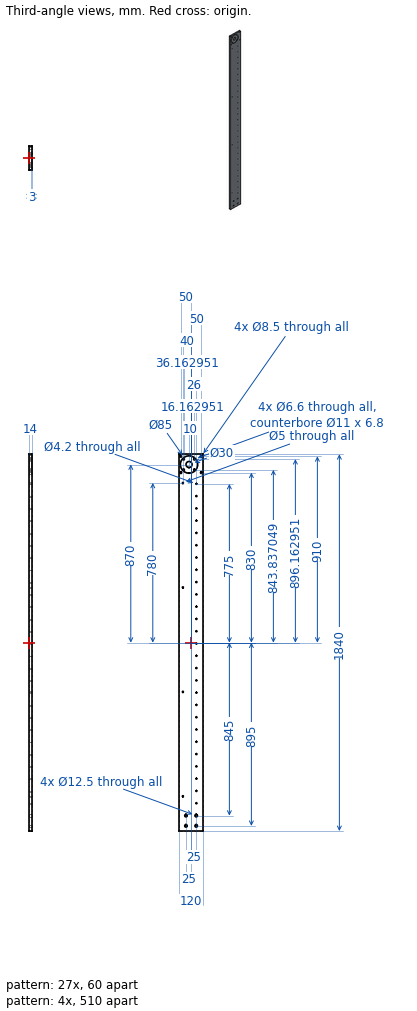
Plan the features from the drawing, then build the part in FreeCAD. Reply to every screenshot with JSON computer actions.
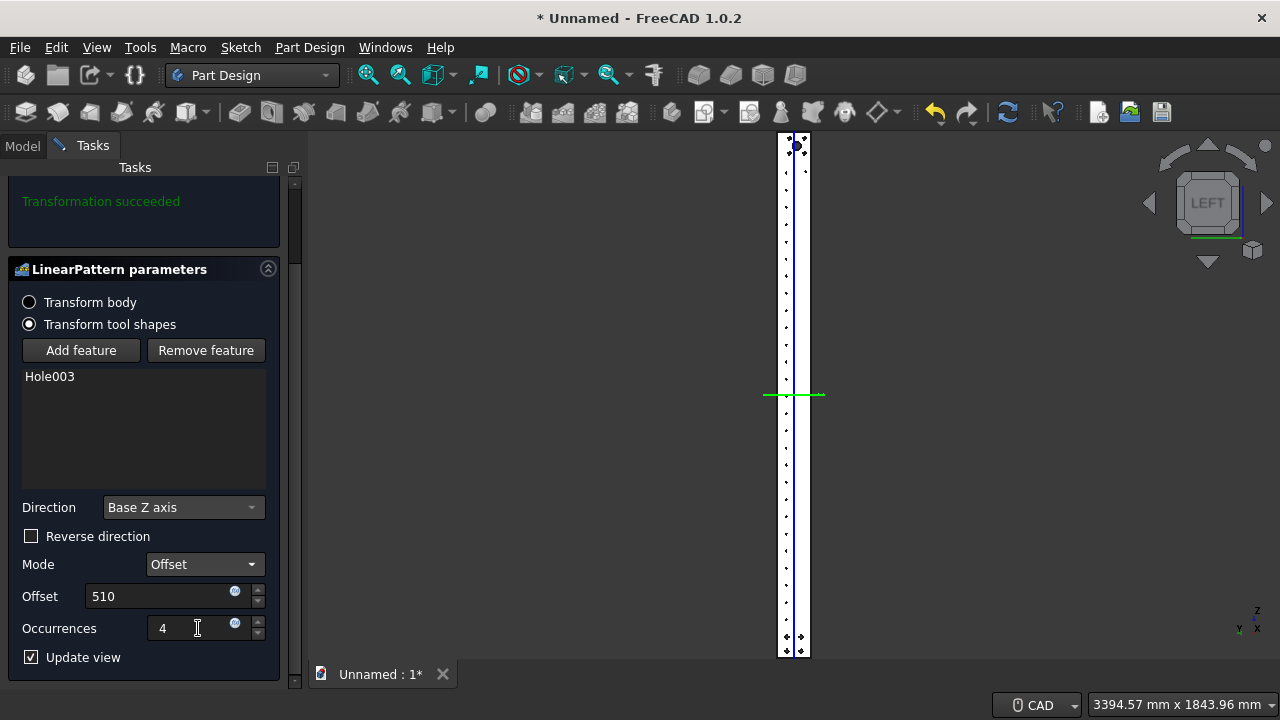
{"action": "left_click", "coordinate": [30, 536]}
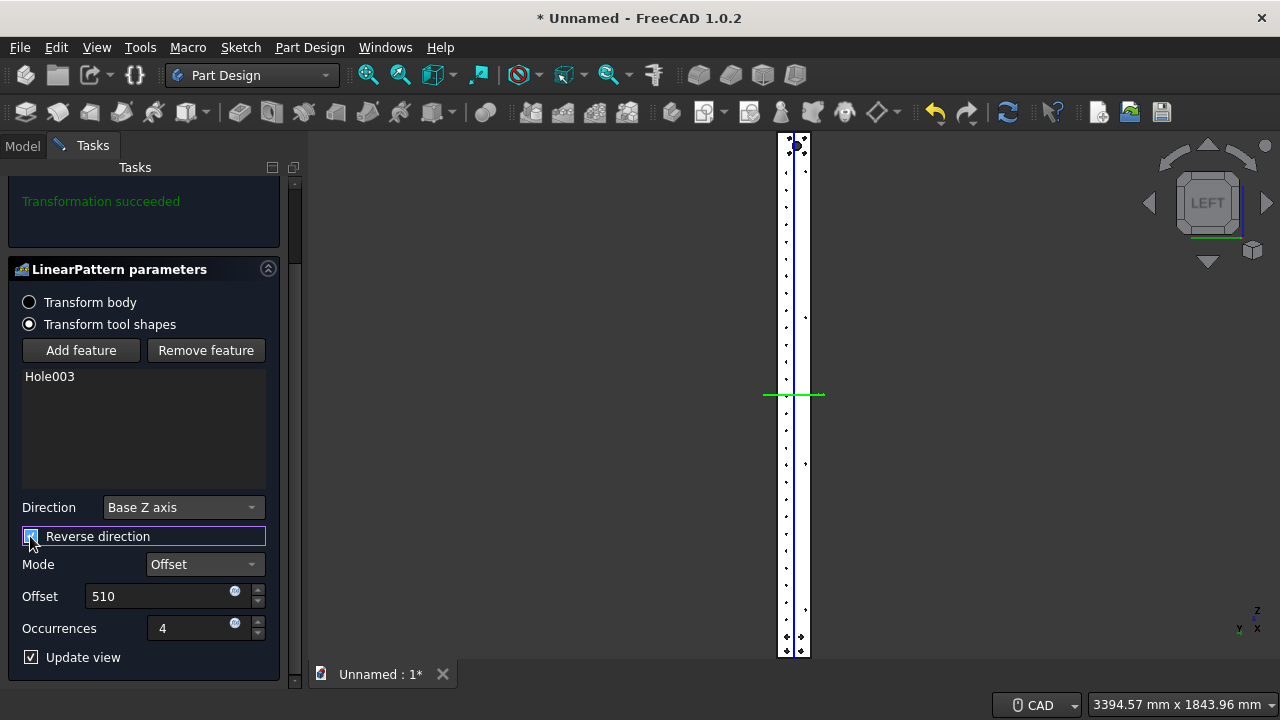
{"action": "scroll", "coordinate": [295, 432], "scroll_direction": "up", "scroll_amount": 3}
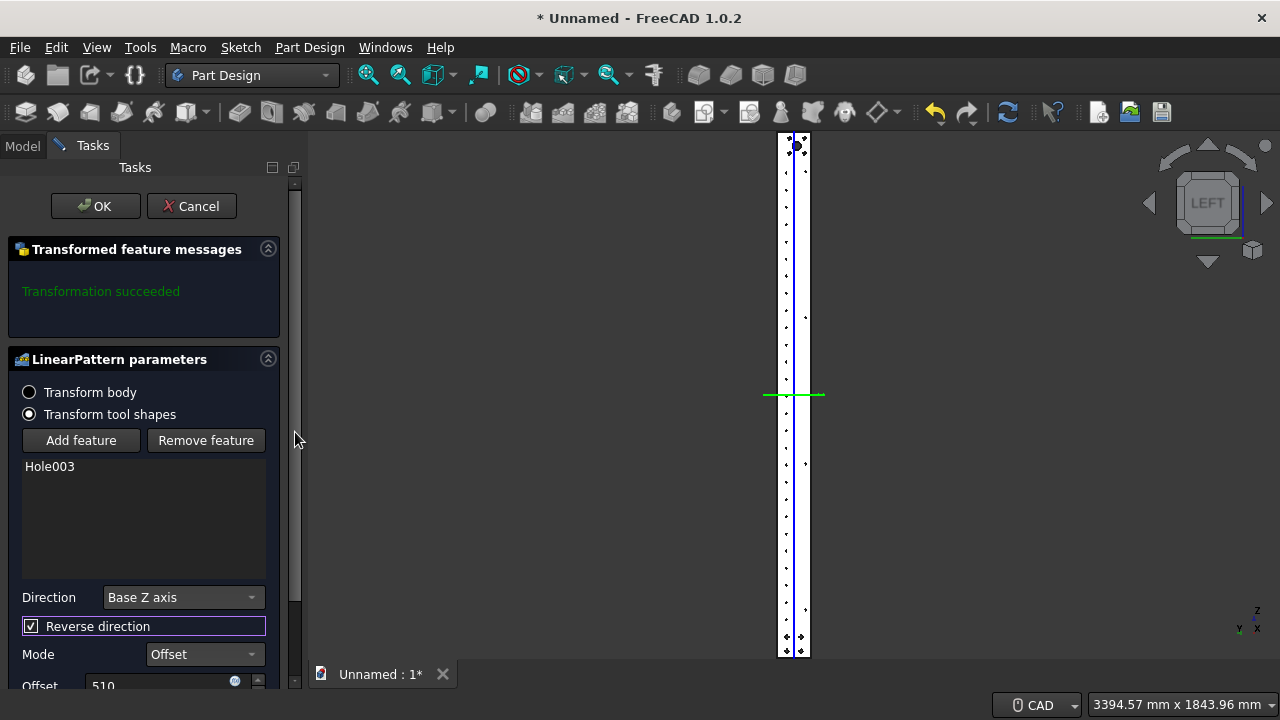
{"action": "left_click", "coordinate": [96, 206]}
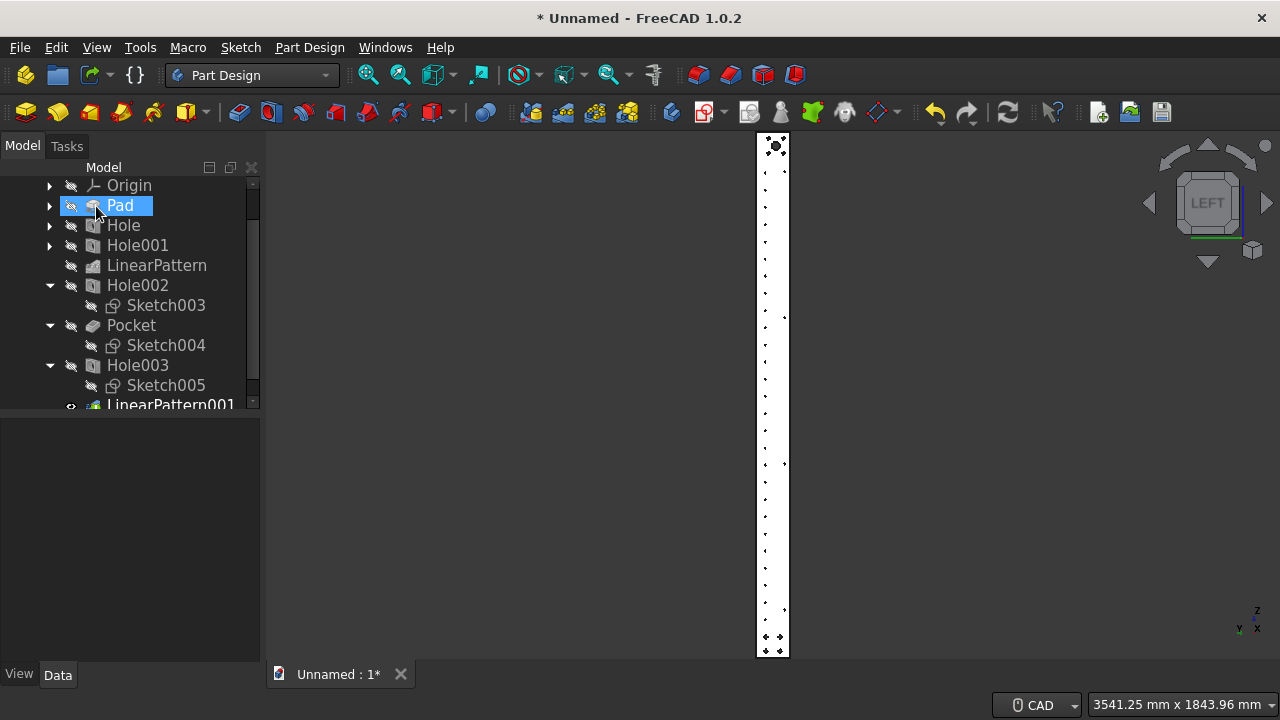
{"action": "key", "text": "0"}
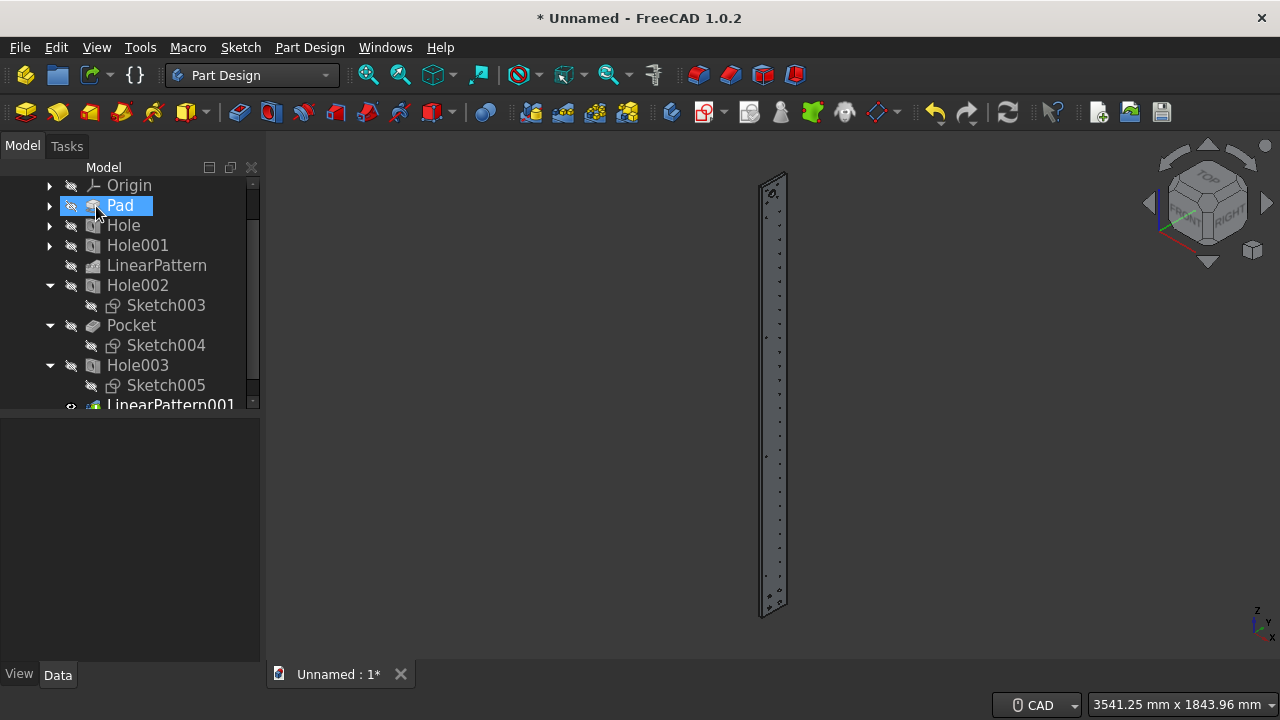
{"action": "left_click", "coordinate": [771, 520]}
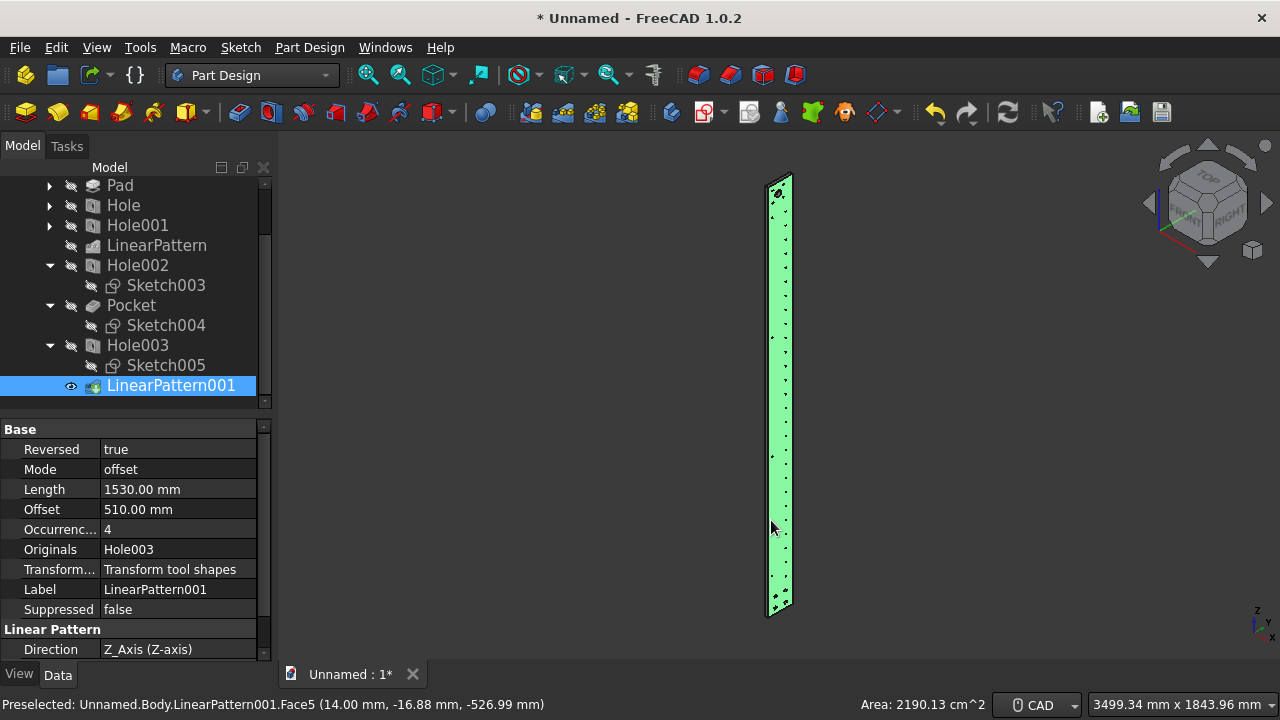
{"action": "left_click", "coordinate": [704, 112]}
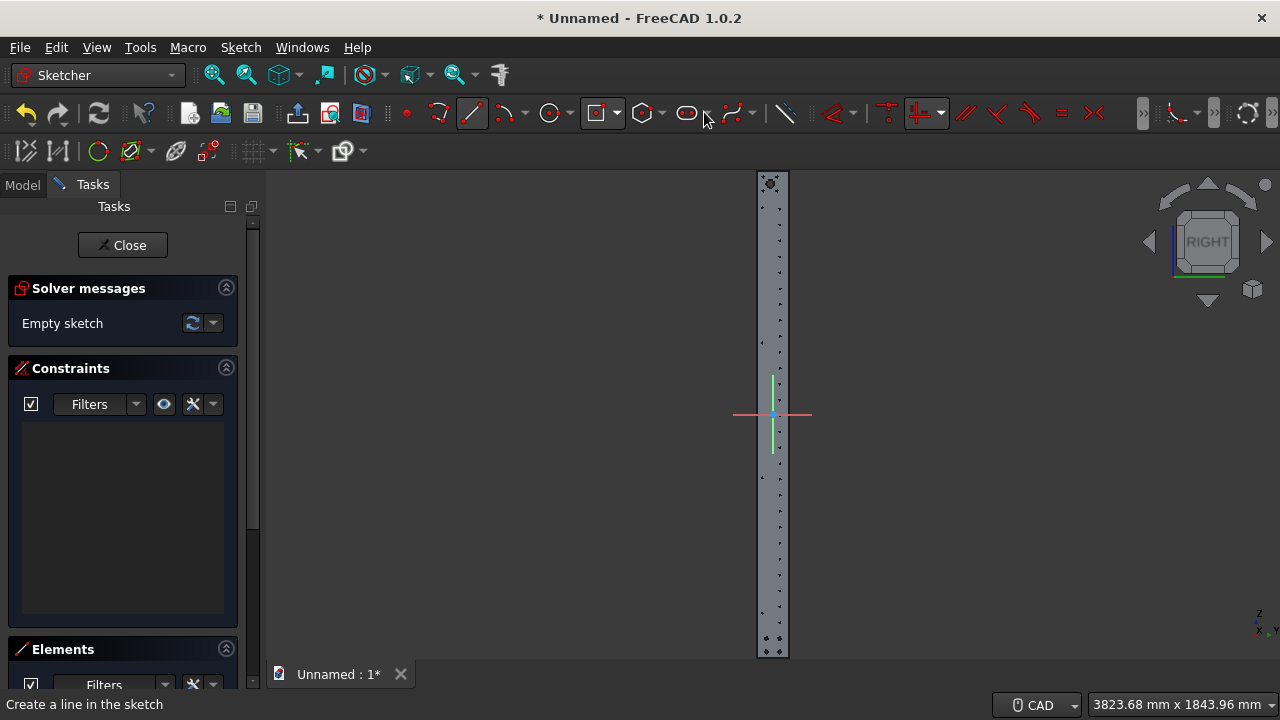
{"action": "scroll", "coordinate": [704, 414], "scroll_direction": "down", "scroll_amount": 5}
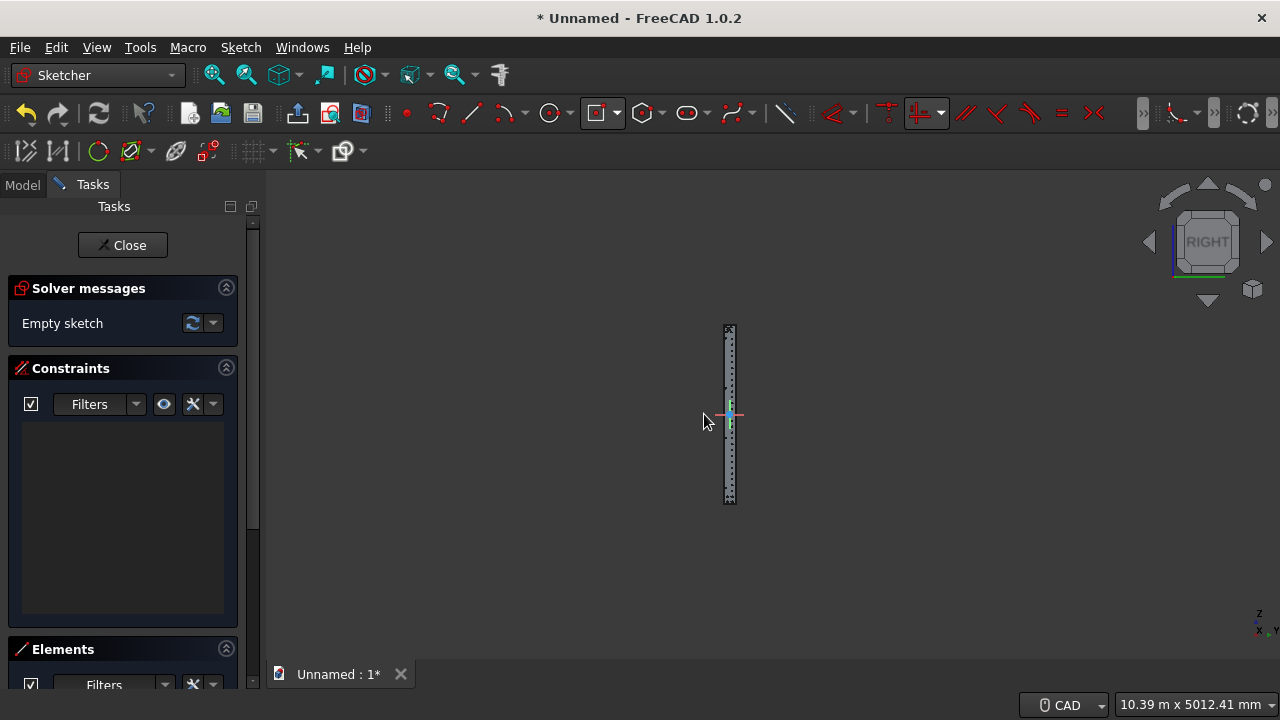
{"action": "scroll", "coordinate": [731, 325], "scroll_direction": "up", "scroll_amount": 15}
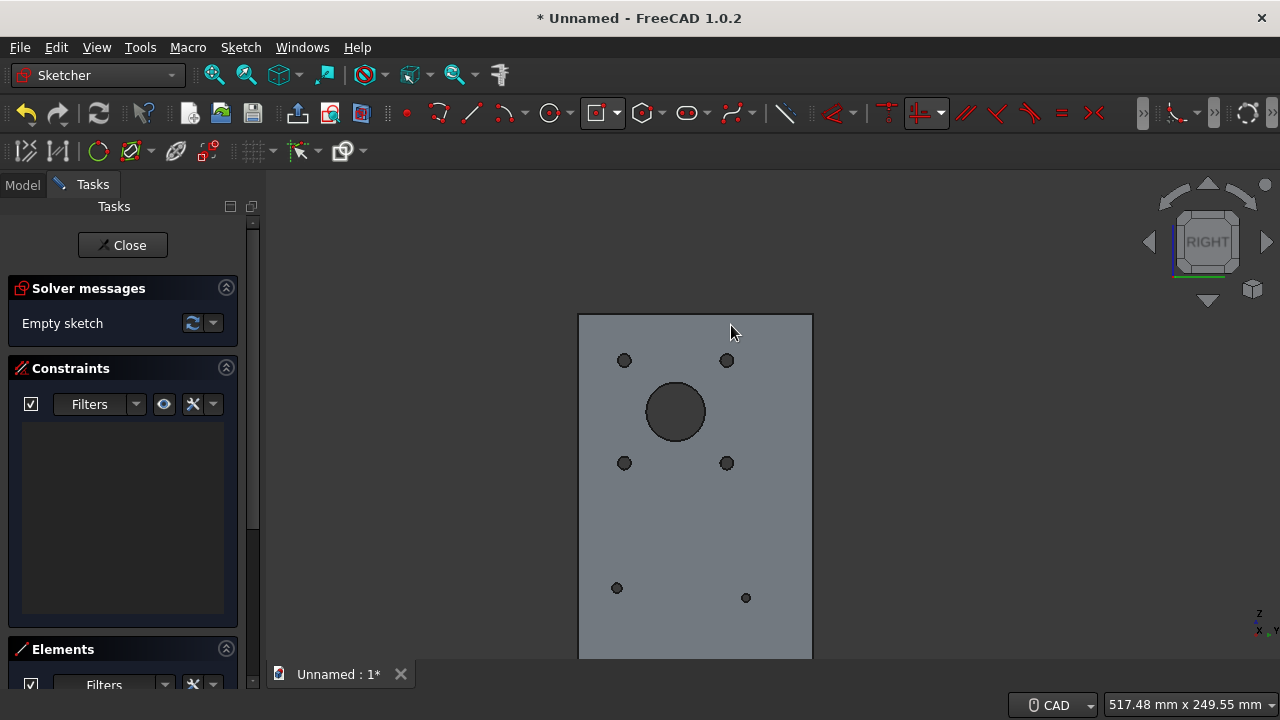
{"action": "scroll", "coordinate": [684, 409], "scroll_direction": "up", "scroll_amount": 3}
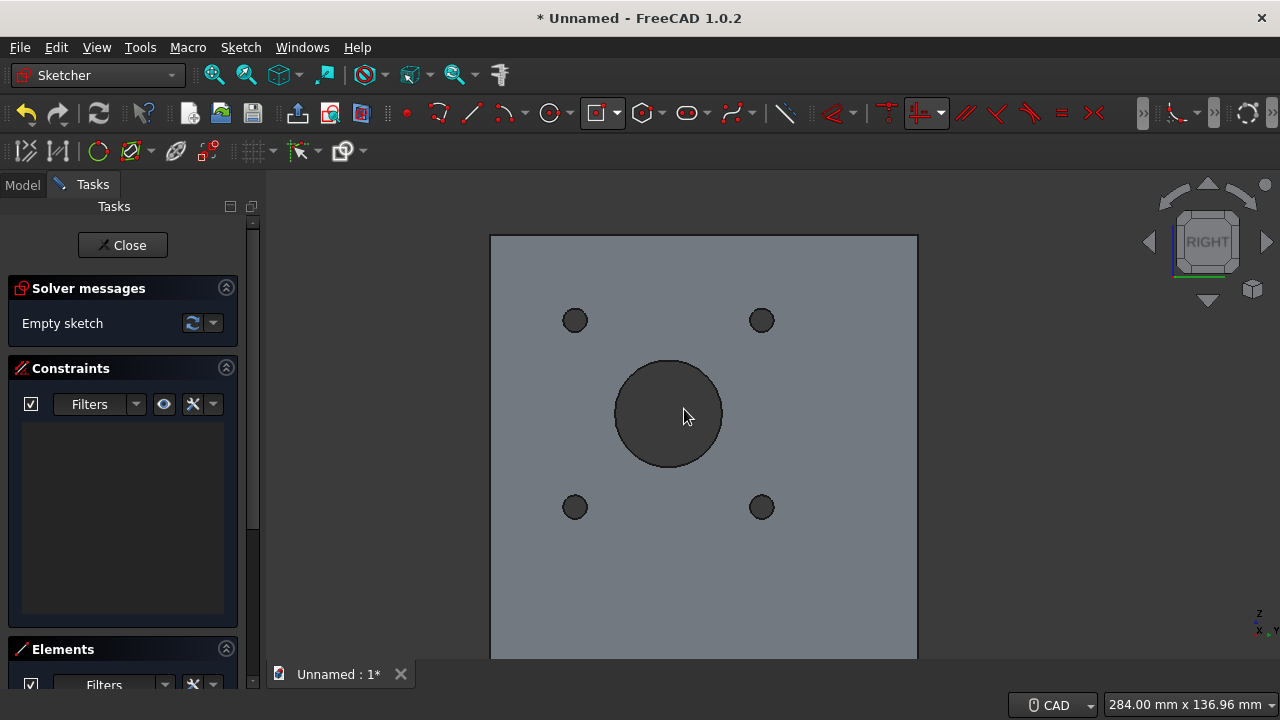
{"action": "left_click", "coordinate": [550, 114]}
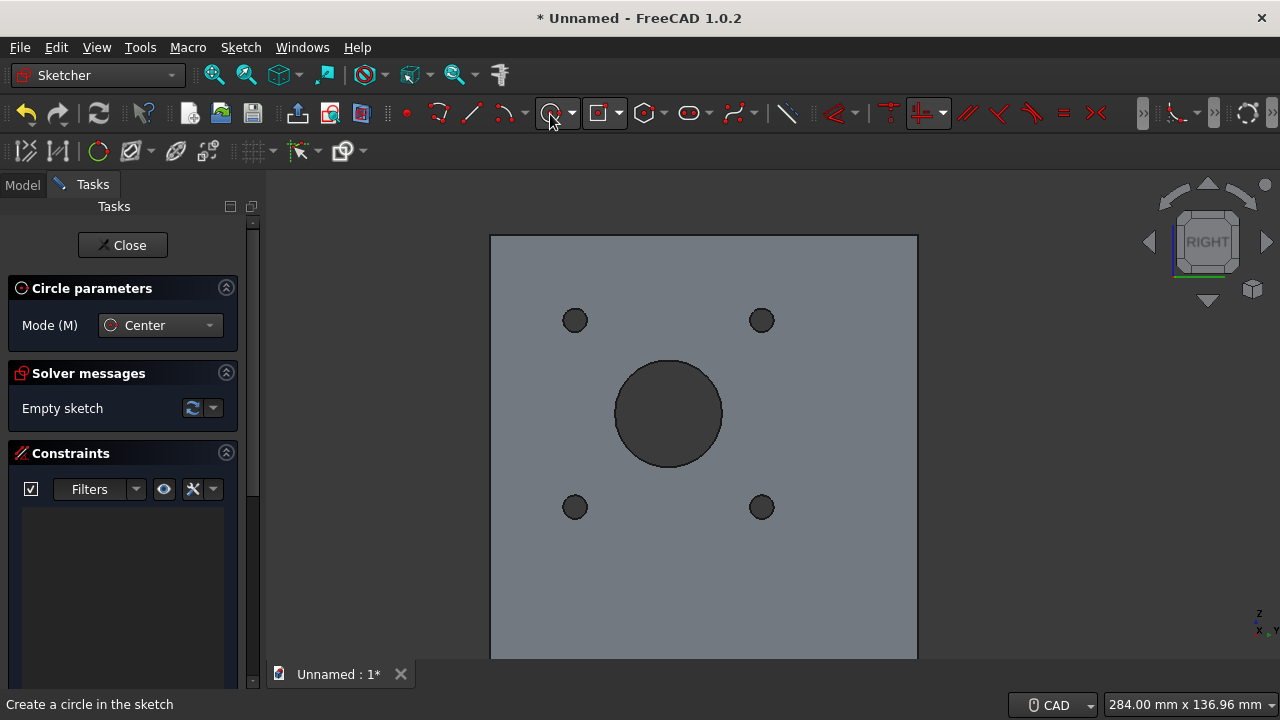
{"action": "scroll", "coordinate": [883, 271], "scroll_direction": "up", "scroll_amount": 3}